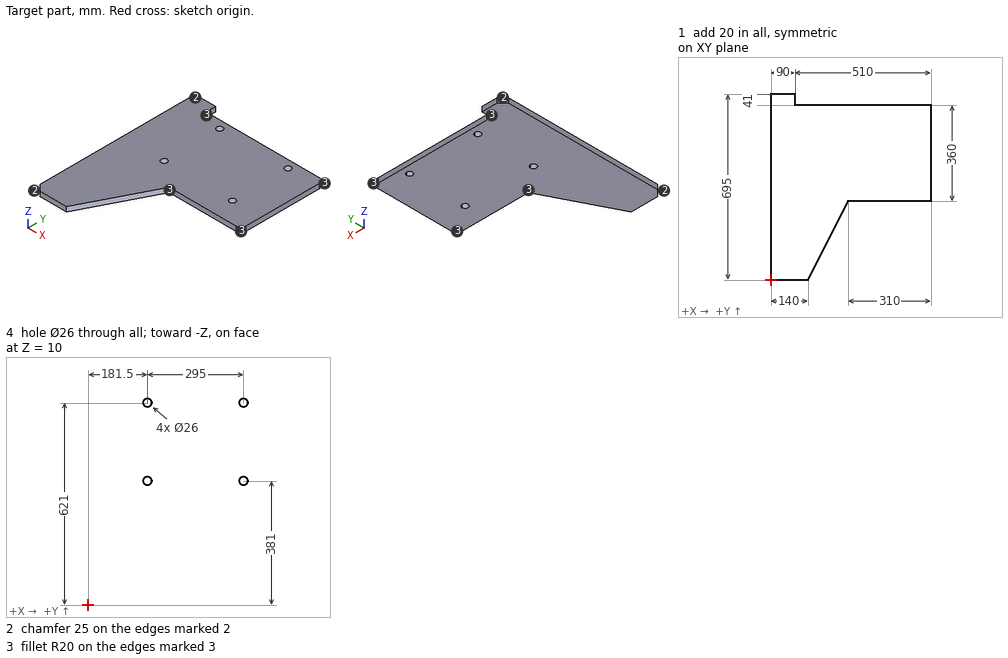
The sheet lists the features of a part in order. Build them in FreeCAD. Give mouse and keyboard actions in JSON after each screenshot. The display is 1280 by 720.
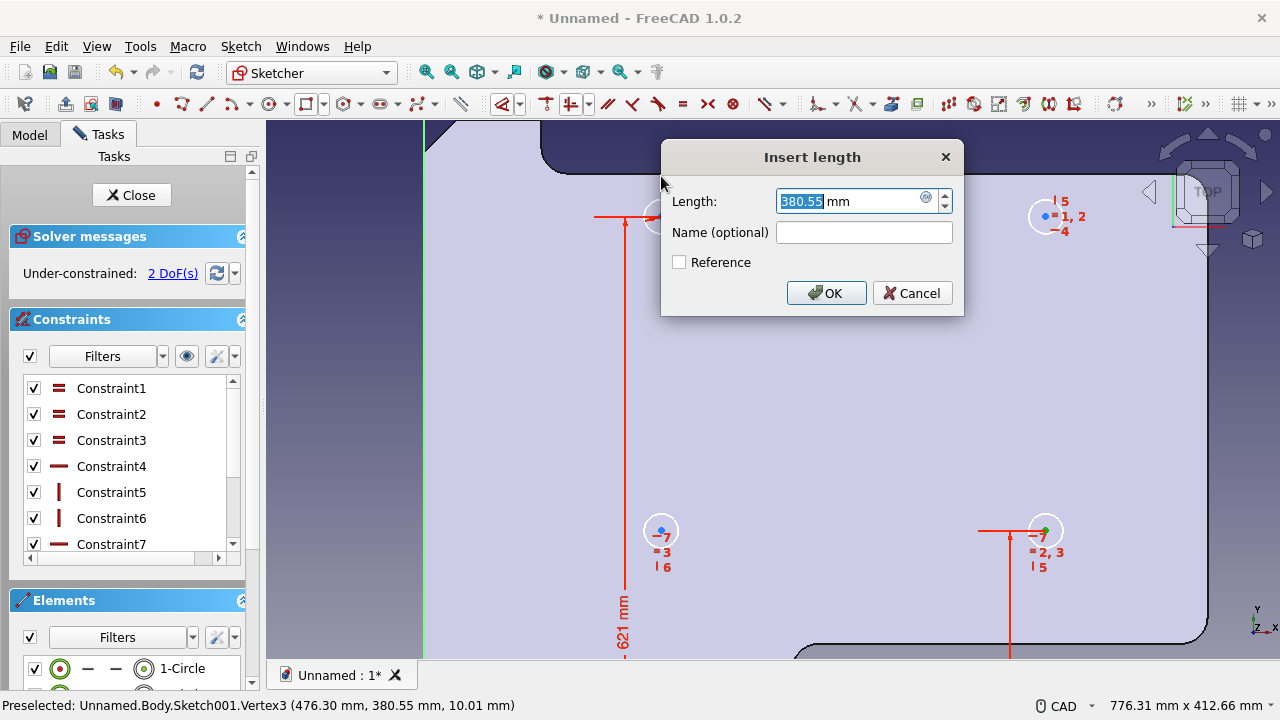
{"action": "type", "text": "381"}
{"action": "key", "text": "Return"}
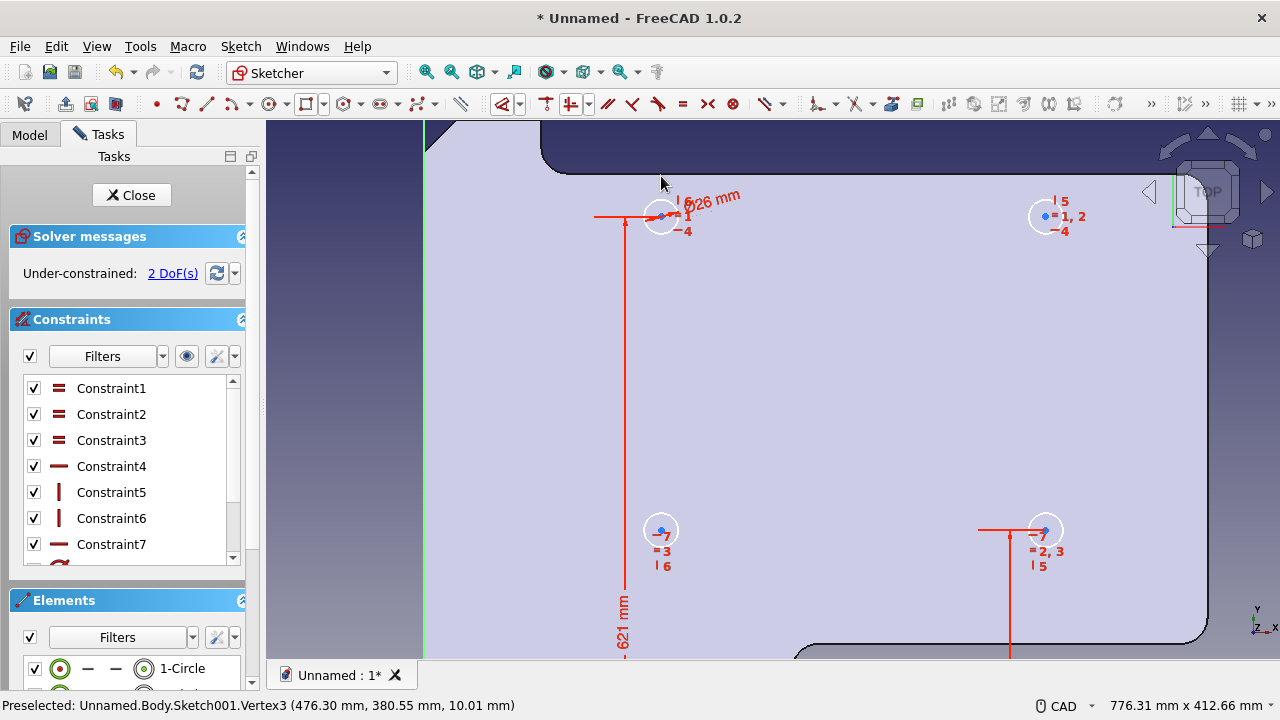
{"action": "left_click", "coordinate": [661, 217]}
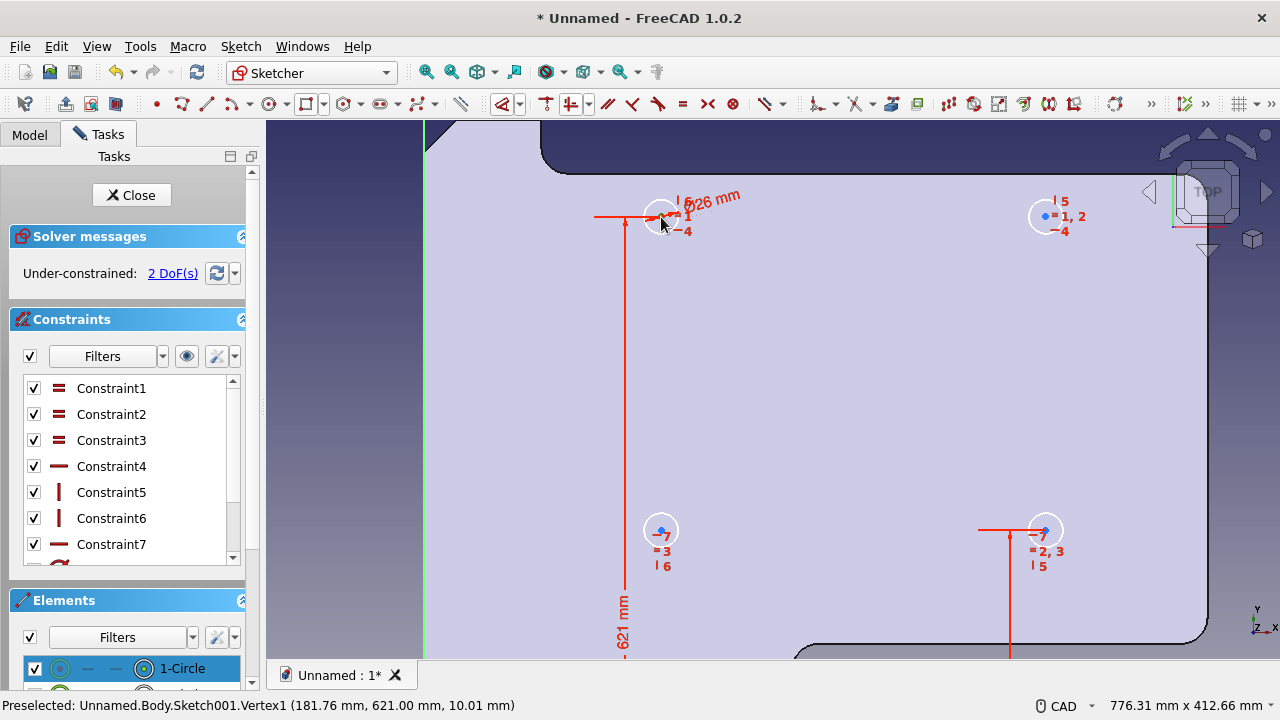
{"action": "left_click", "coordinate": [1046, 217]}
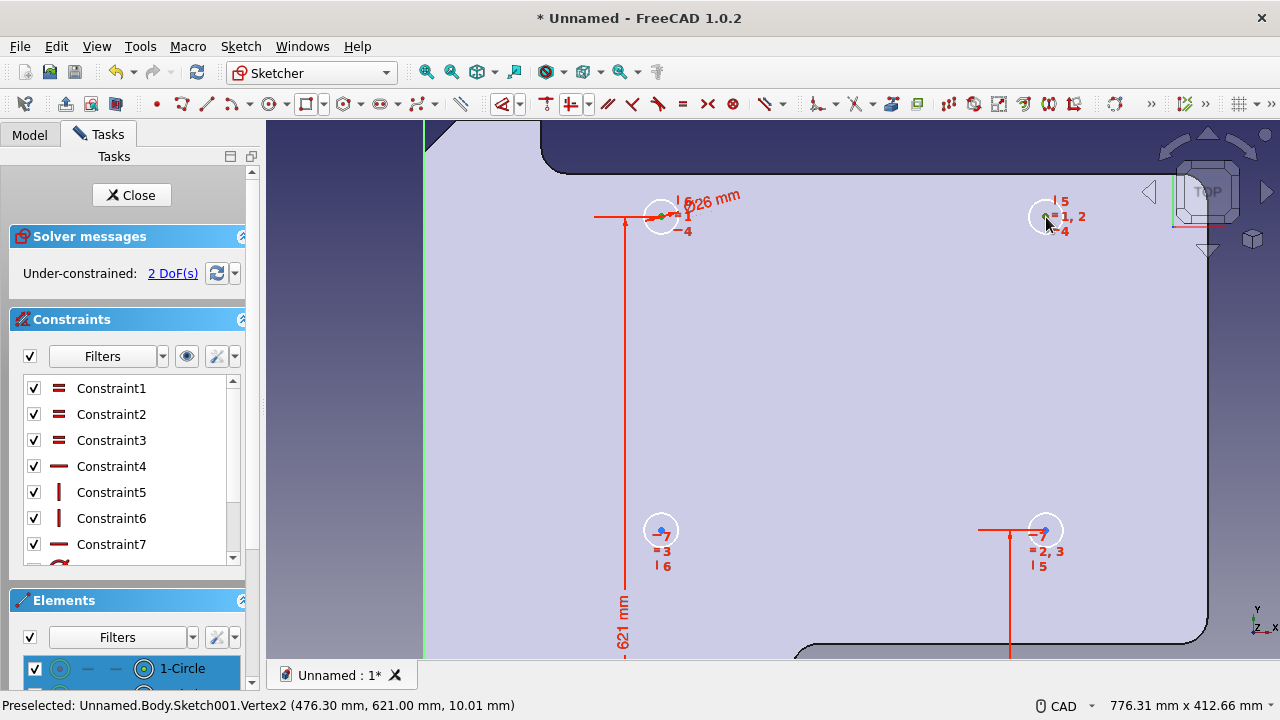
{"action": "left_click", "coordinate": [520, 104]}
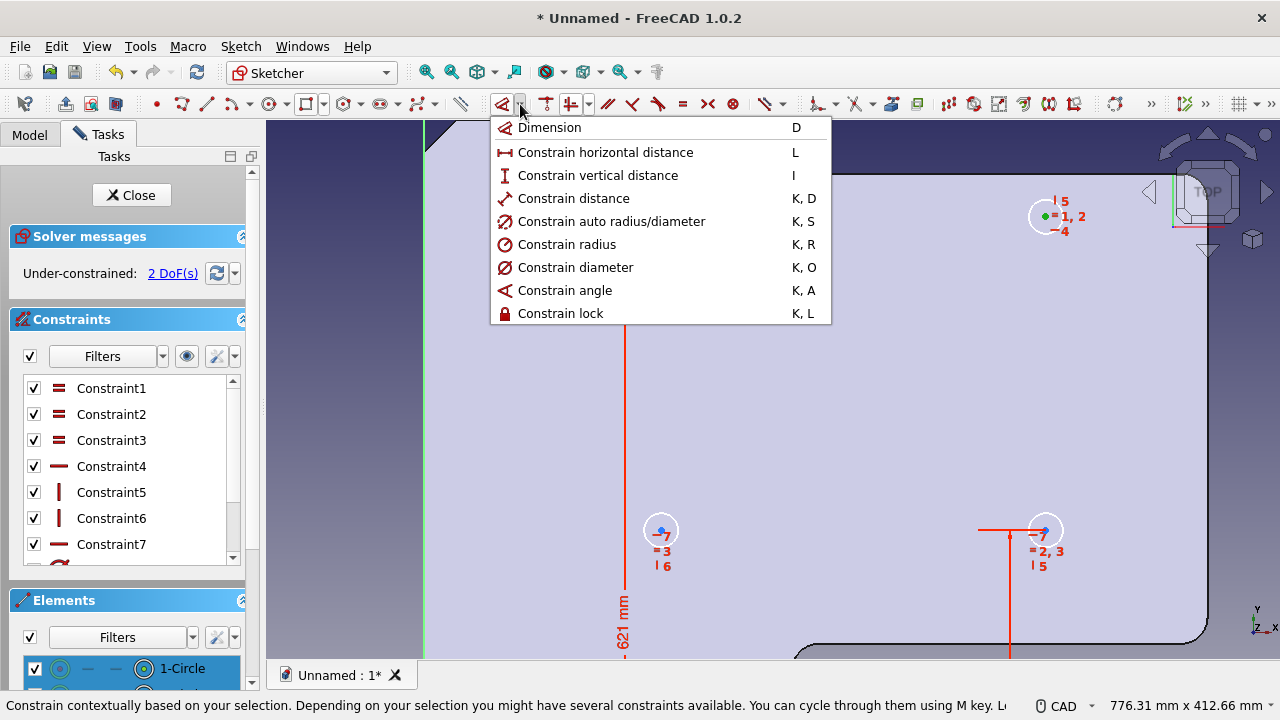
{"action": "left_click", "coordinate": [661, 152]}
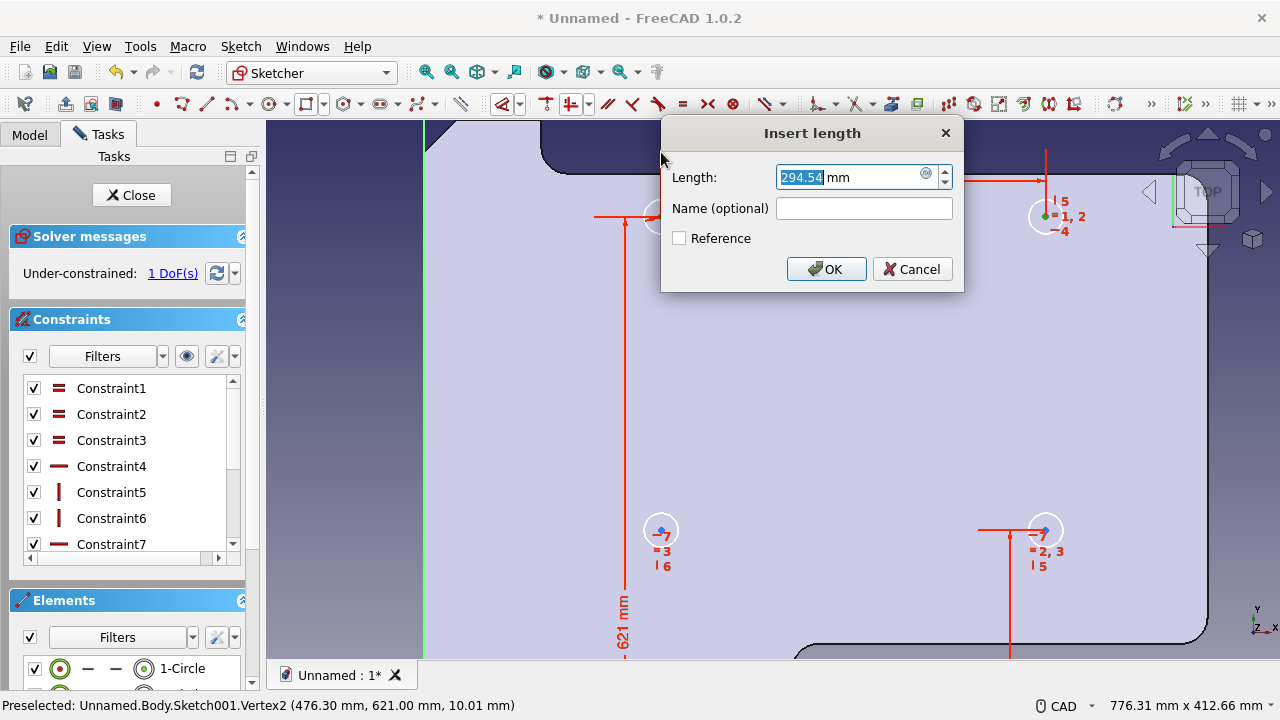
{"action": "type", "text": "295"}
{"action": "key", "text": "Return"}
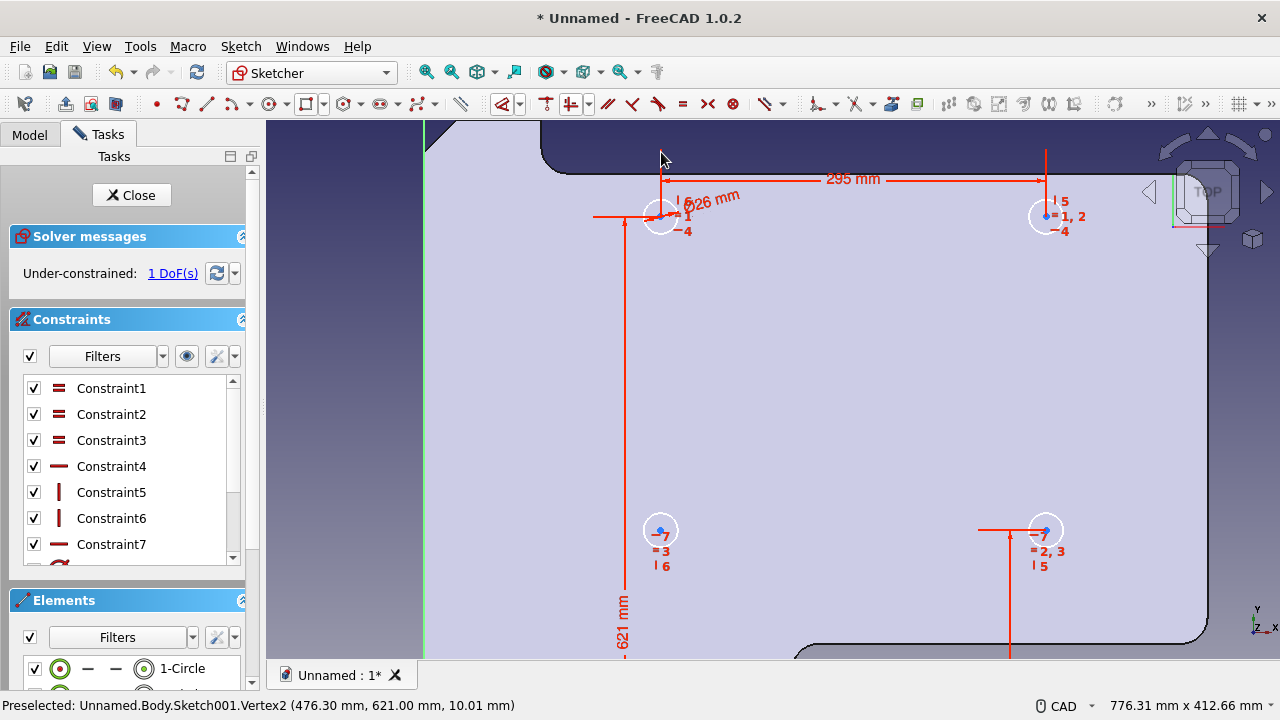
{"action": "left_click", "coordinate": [661, 217]}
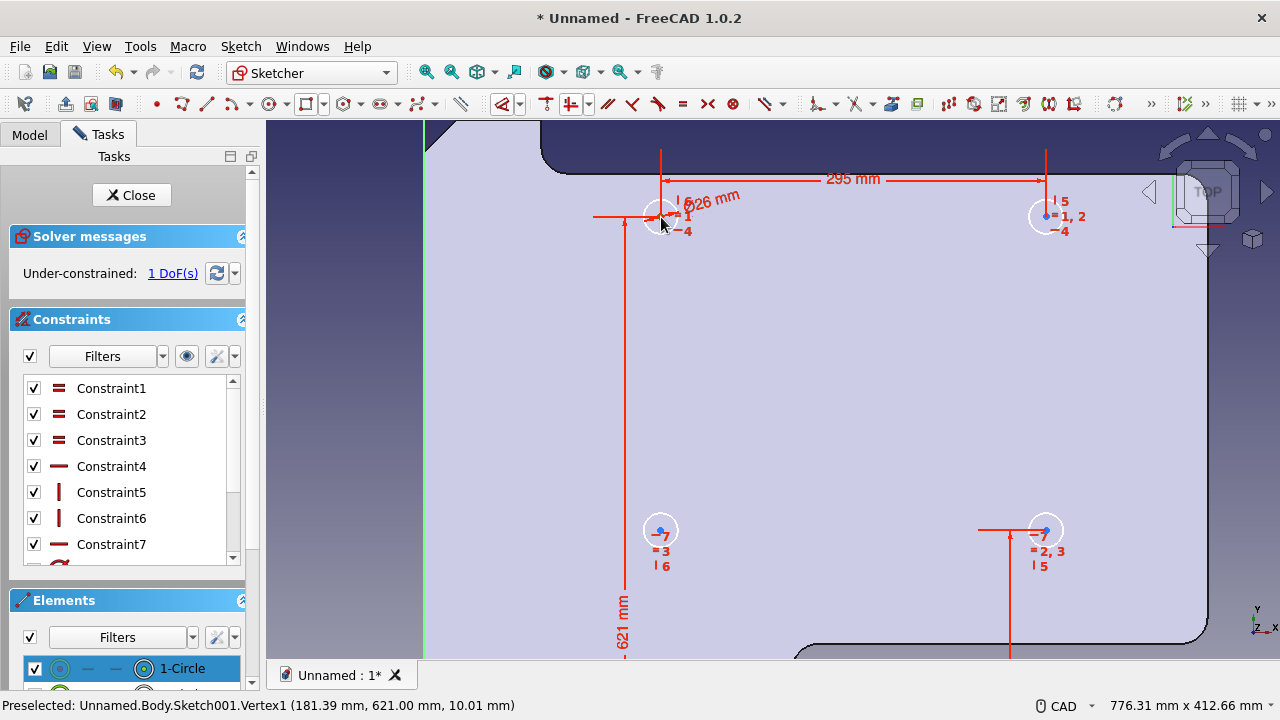
{"action": "left_click", "coordinate": [520, 104]}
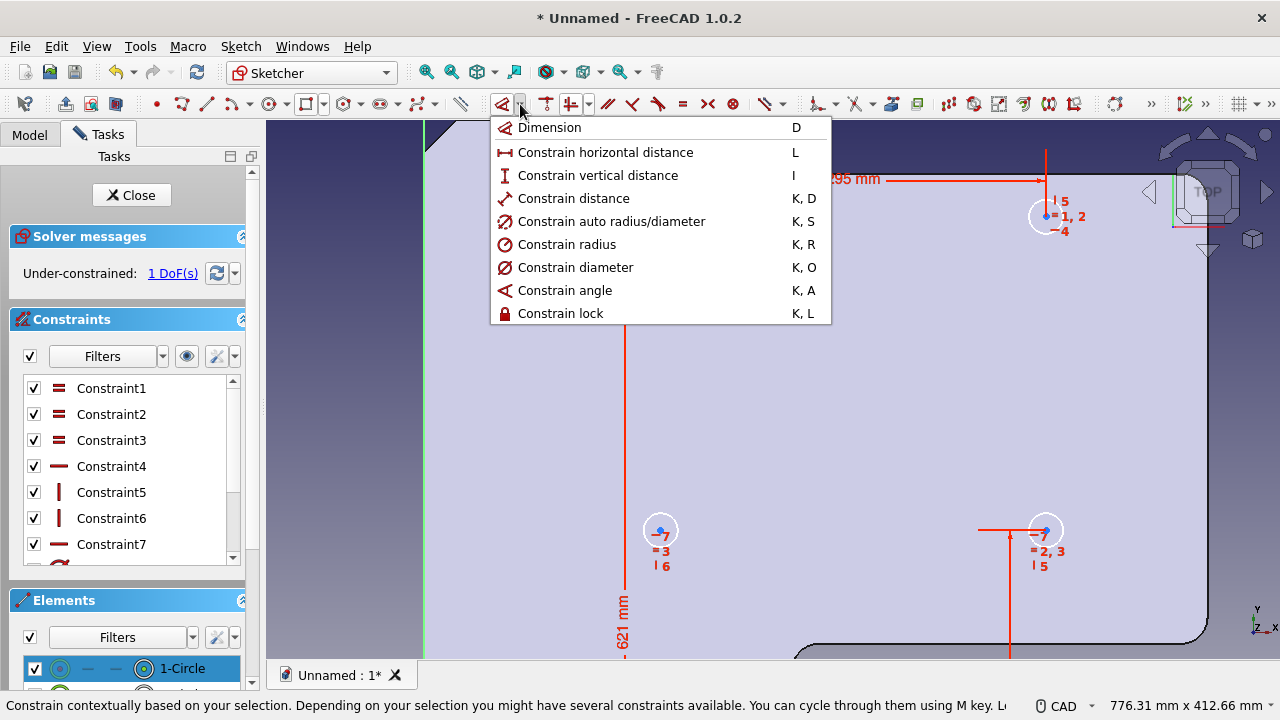
{"action": "left_click", "coordinate": [661, 152]}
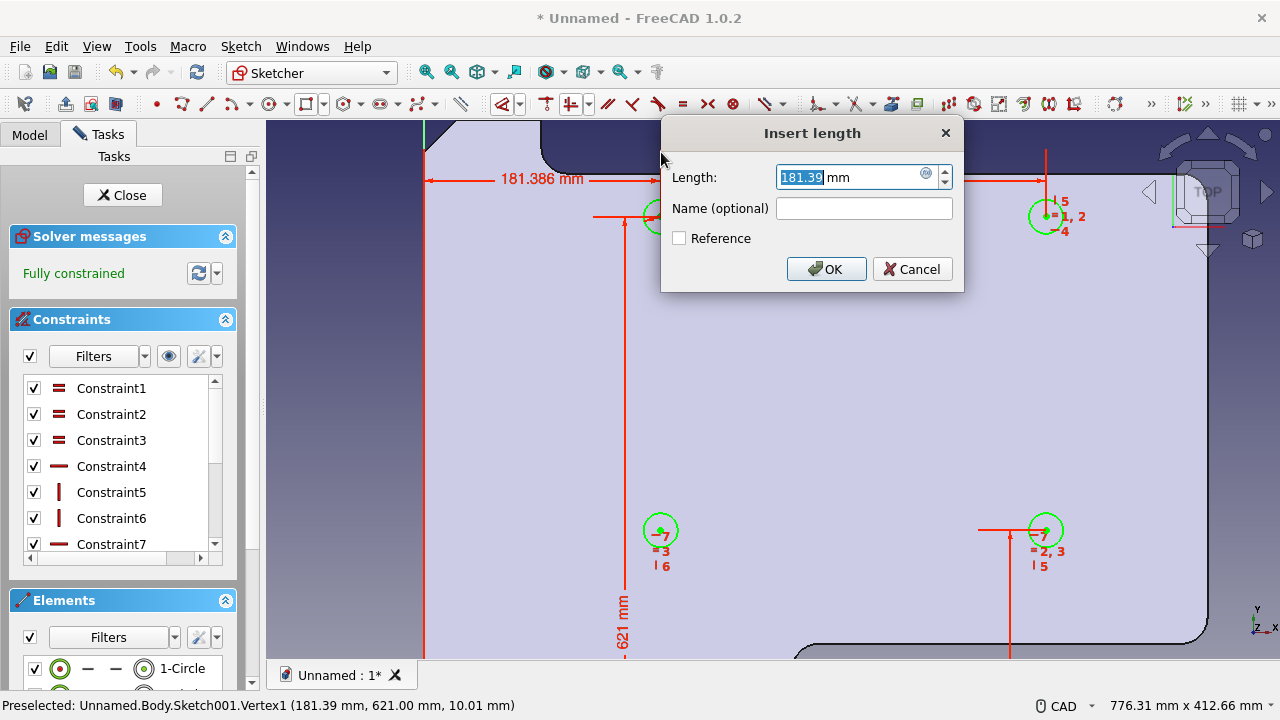
{"action": "type", "text": "181.5"}
{"action": "key", "text": "Return"}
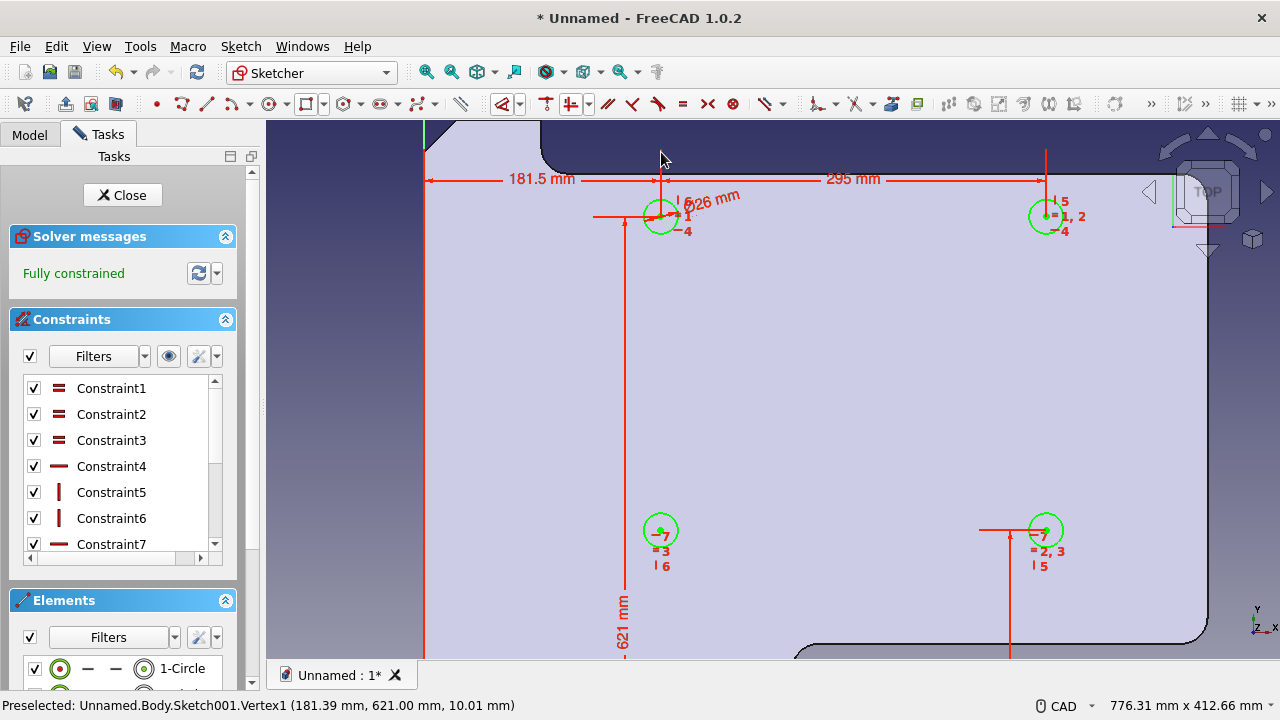
{"action": "left_click", "coordinate": [123, 195]}